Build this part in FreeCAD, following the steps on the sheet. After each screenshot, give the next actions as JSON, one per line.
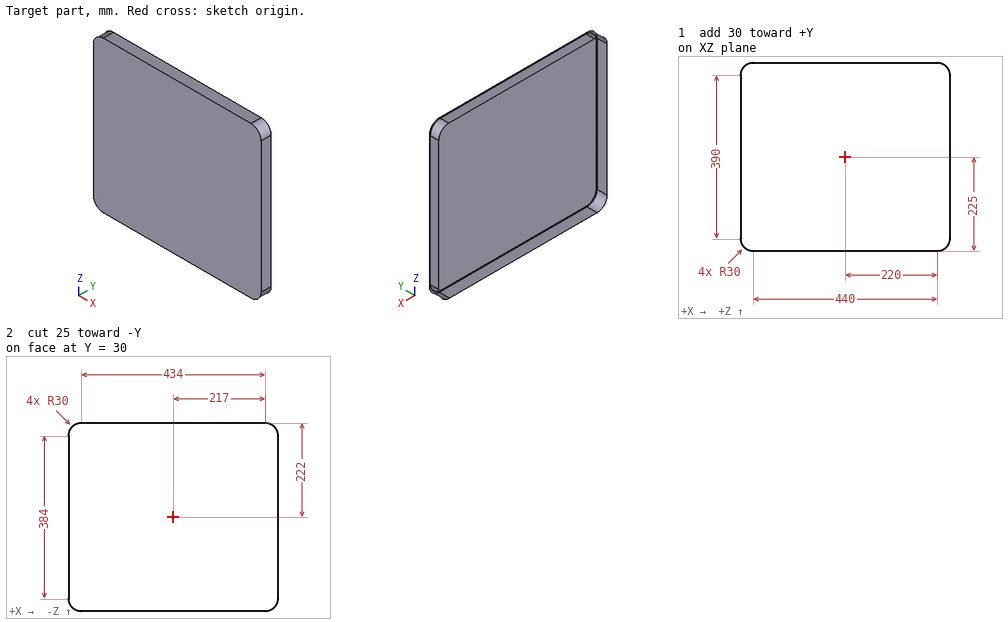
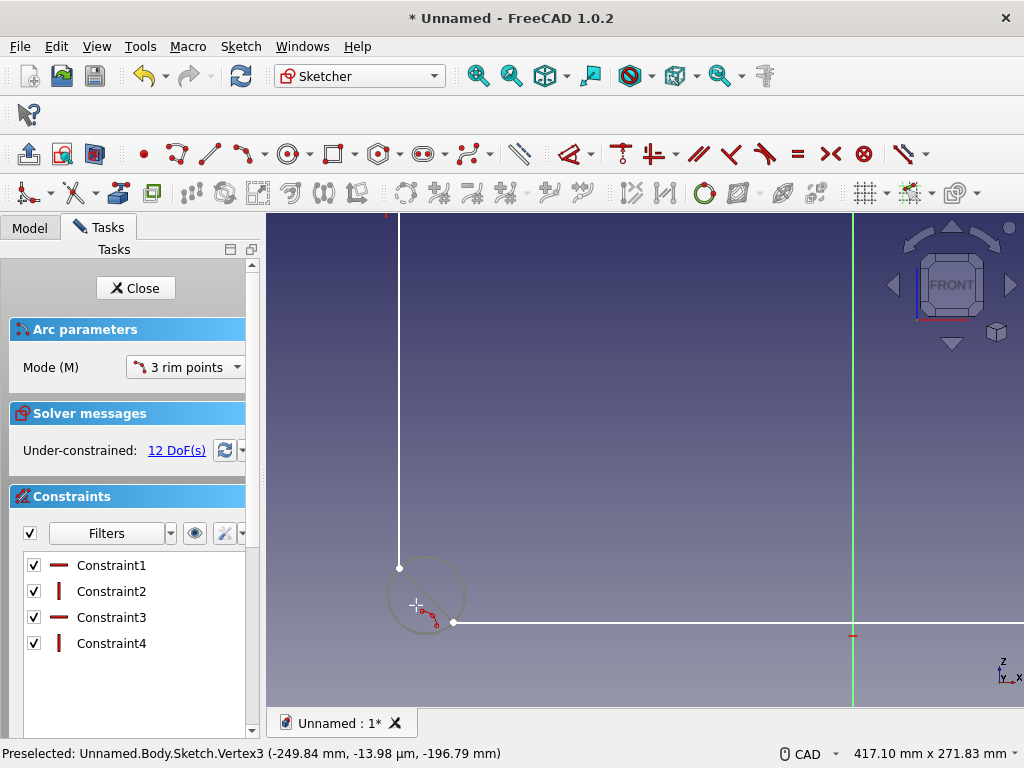
{"action": "left_click", "coordinate": [415, 604]}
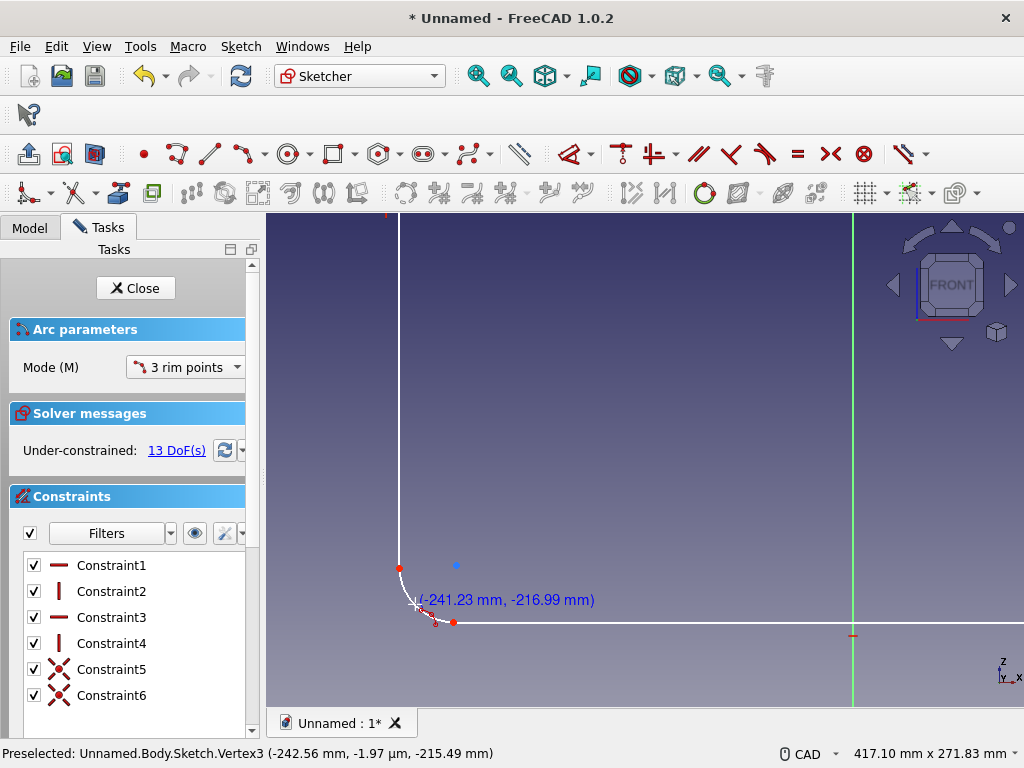
{"action": "scroll", "coordinate": [415, 605], "scroll_direction": "down", "scroll_amount": 5}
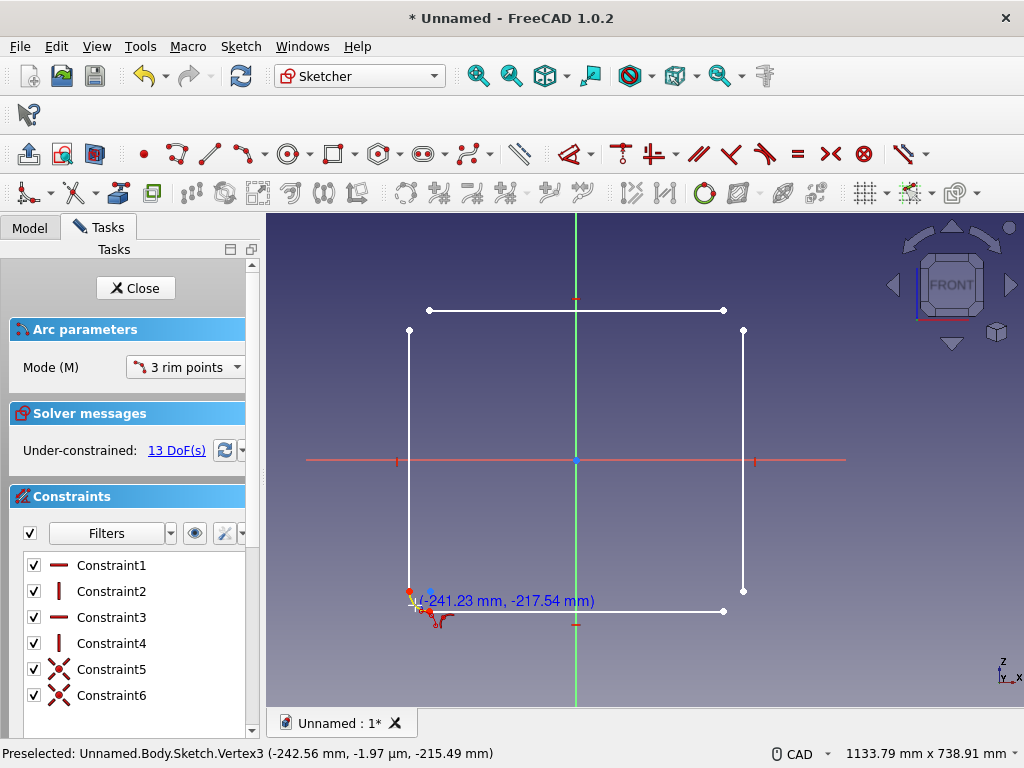
{"action": "left_click", "coordinate": [409, 331]}
{"action": "left_click", "coordinate": [429, 311]}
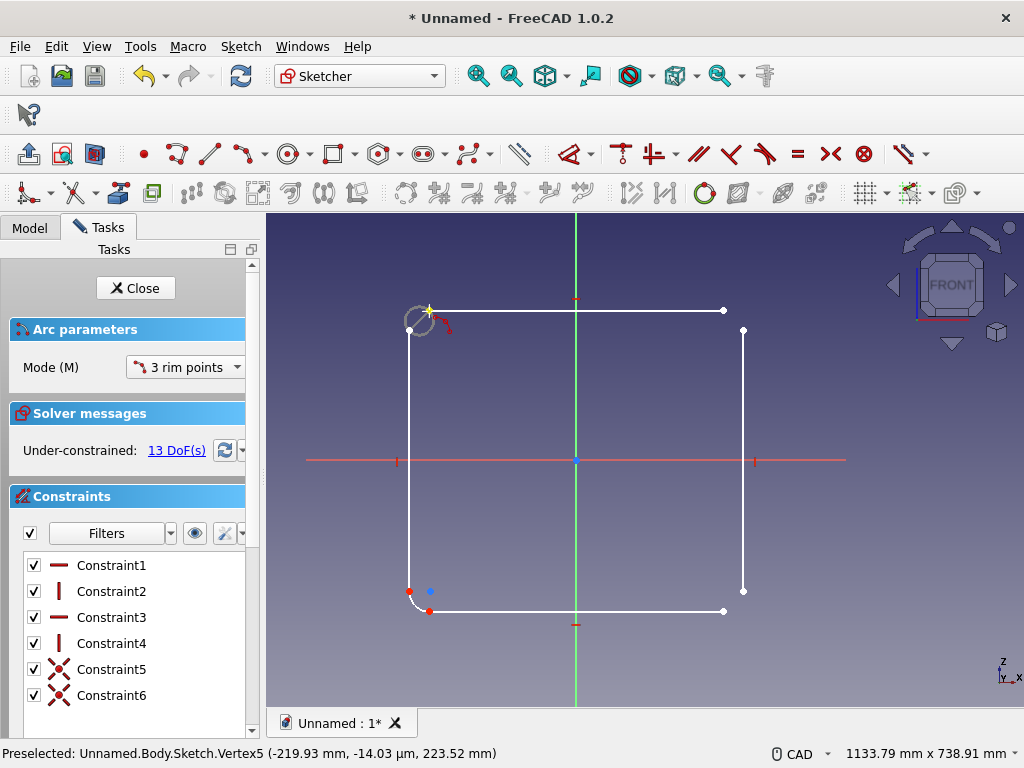
{"action": "scroll", "coordinate": [415, 316], "scroll_direction": "up", "scroll_amount": 5}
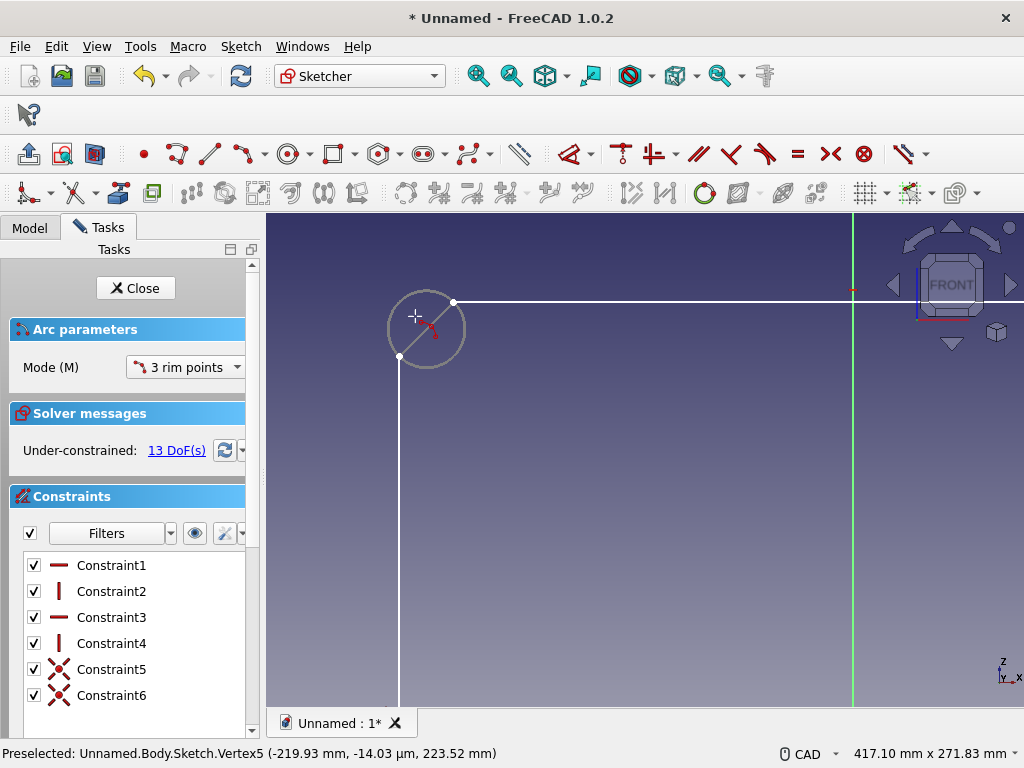
{"action": "left_click", "coordinate": [415, 315]}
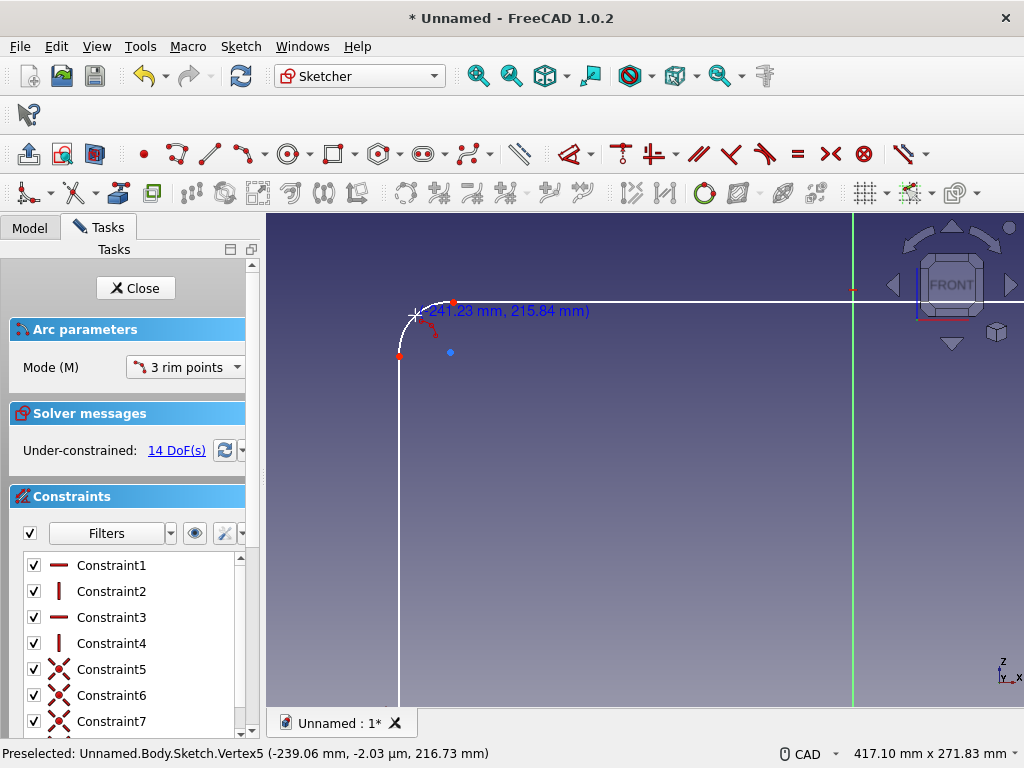
{"action": "scroll", "coordinate": [415, 316], "scroll_direction": "down", "scroll_amount": 5}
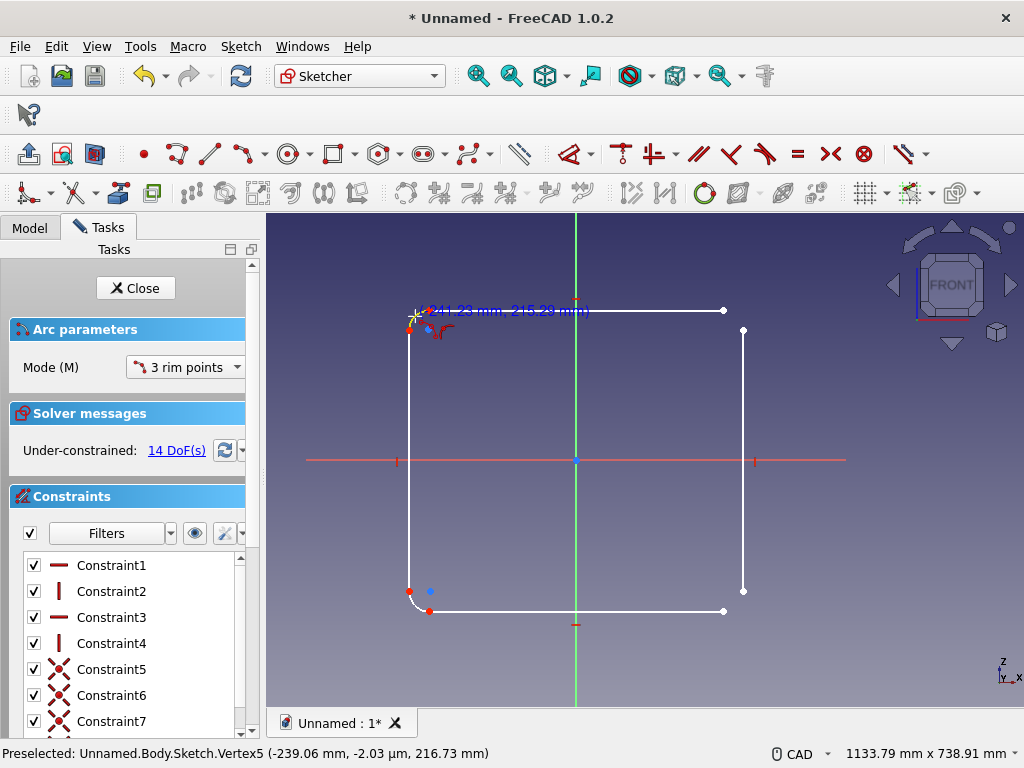
{"action": "left_click", "coordinate": [723, 311]}
{"action": "left_click", "coordinate": [743, 331]}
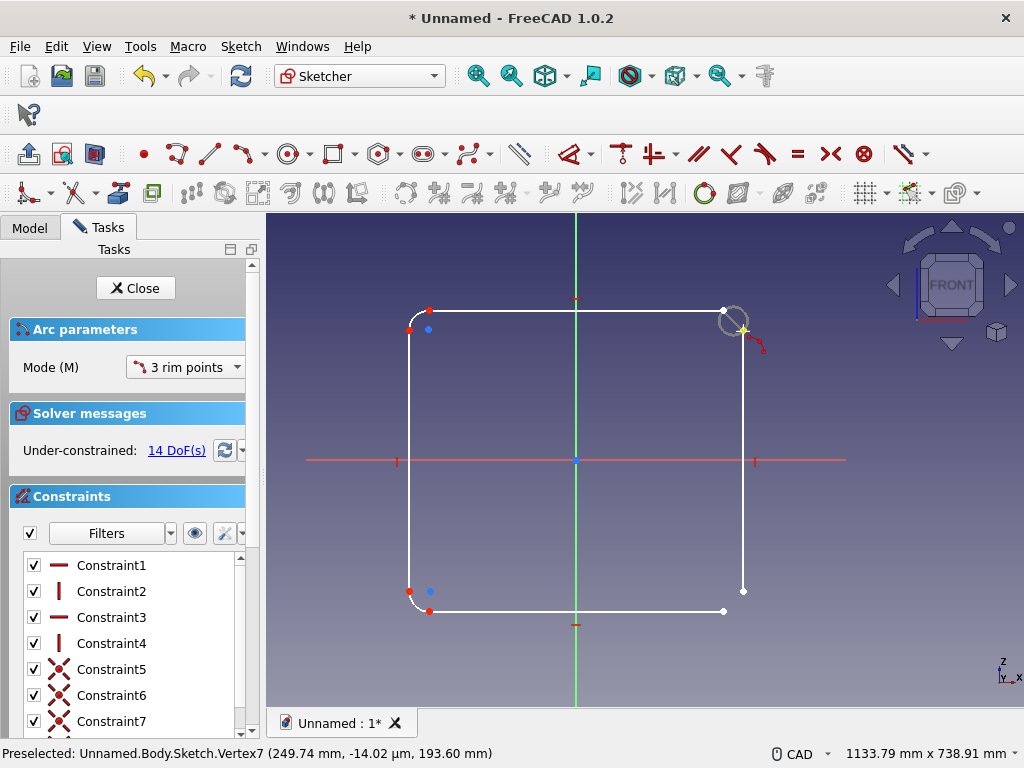
{"action": "scroll", "coordinate": [738, 316], "scroll_direction": "up", "scroll_amount": 5}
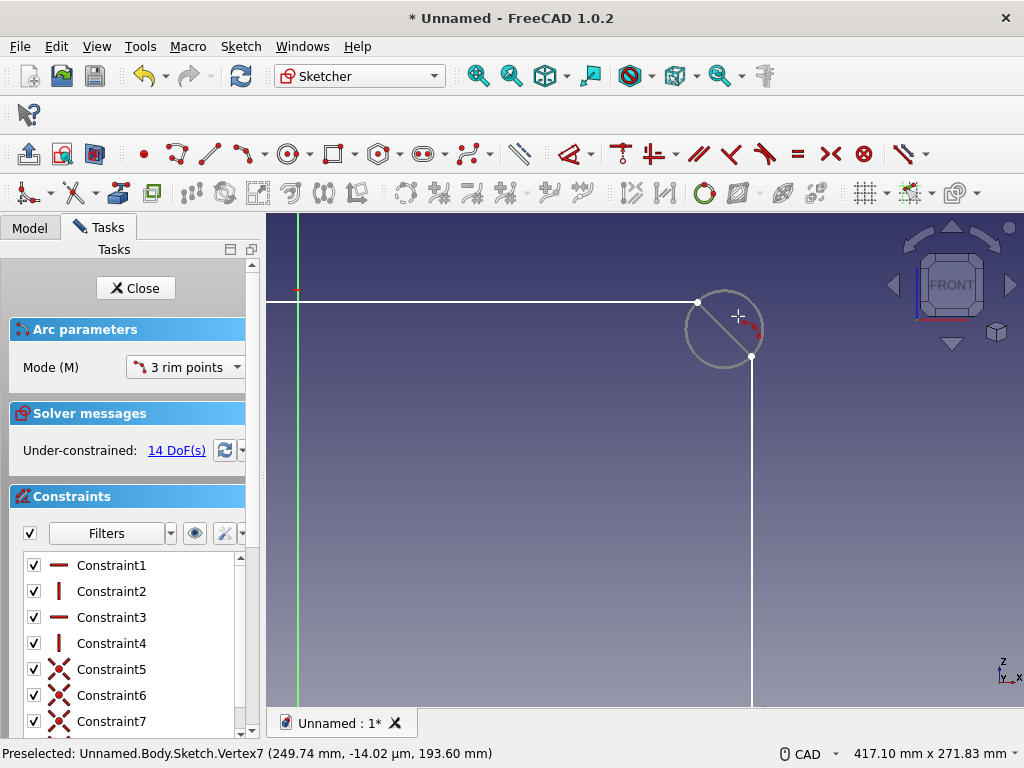
{"action": "left_click", "coordinate": [736, 315]}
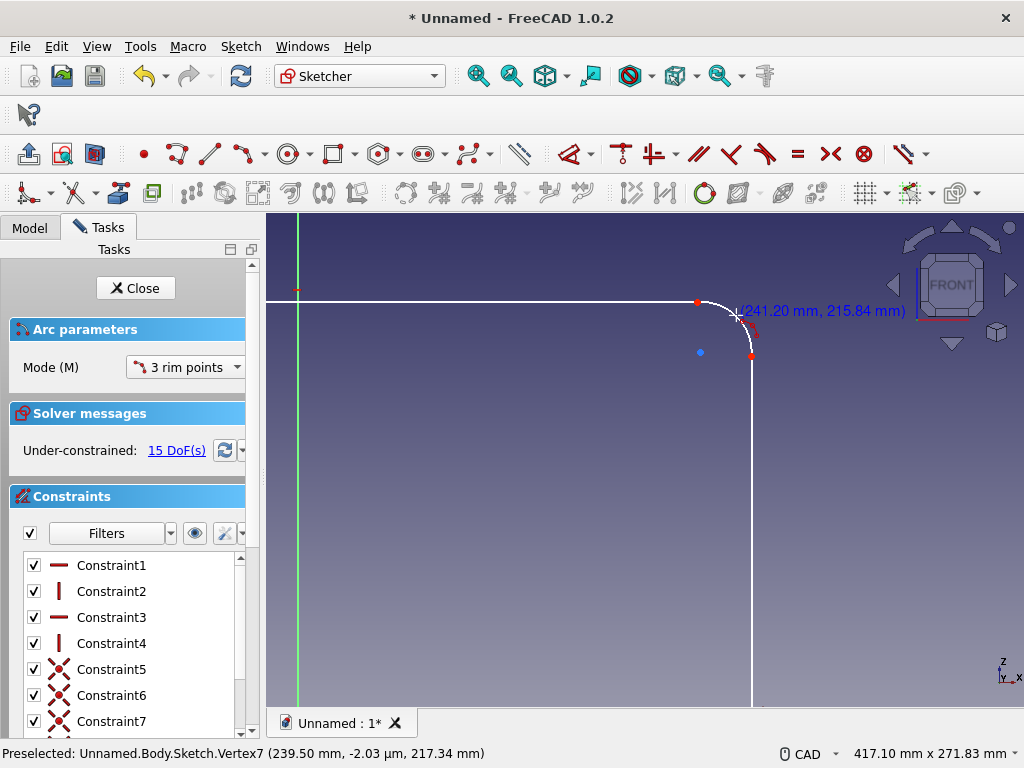
{"action": "scroll", "coordinate": [739, 316], "scroll_direction": "down", "scroll_amount": 5}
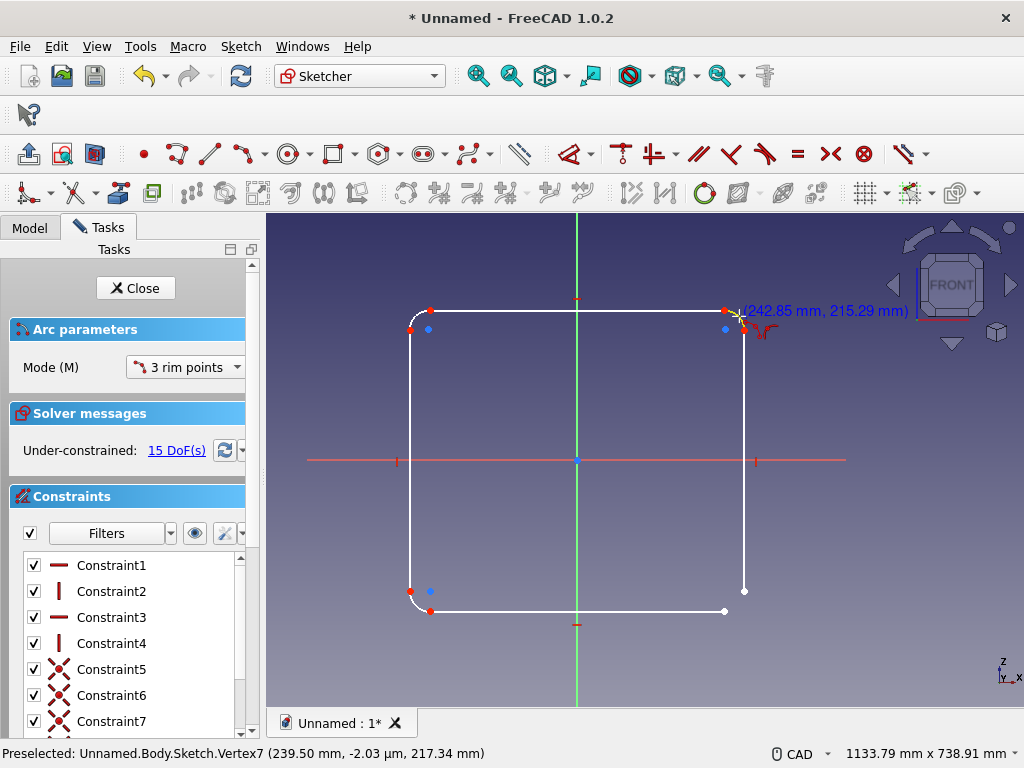
{"action": "left_click", "coordinate": [744, 592]}
{"action": "left_click", "coordinate": [724, 612]}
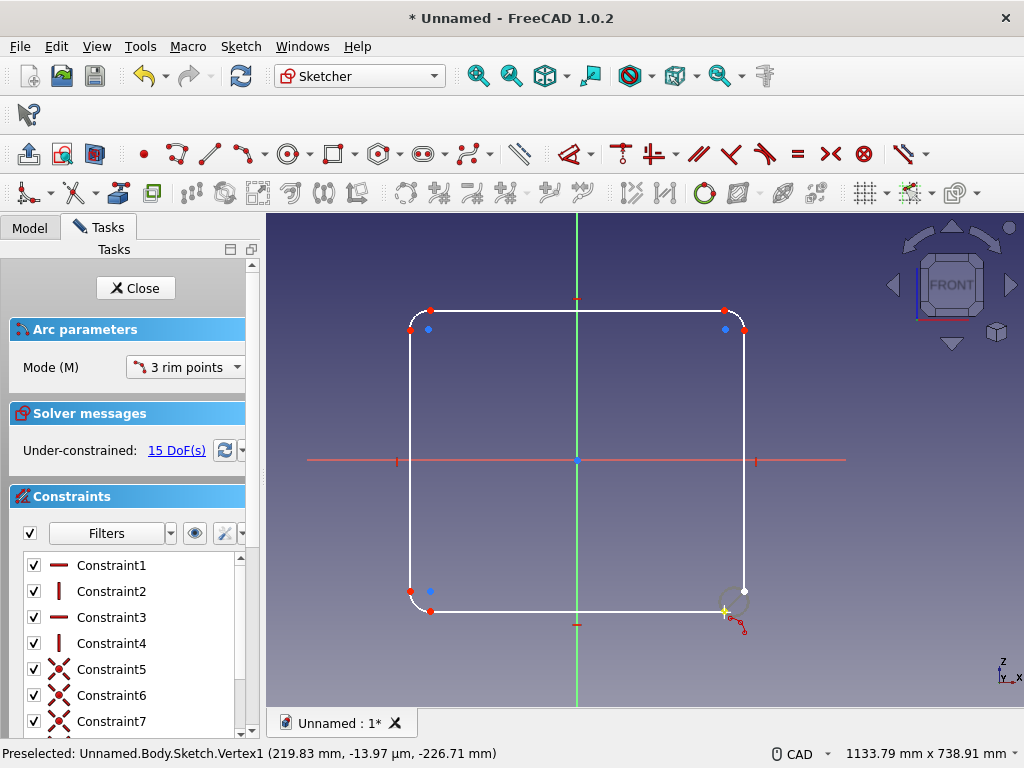
{"action": "scroll", "coordinate": [738, 605], "scroll_direction": "up", "scroll_amount": 5}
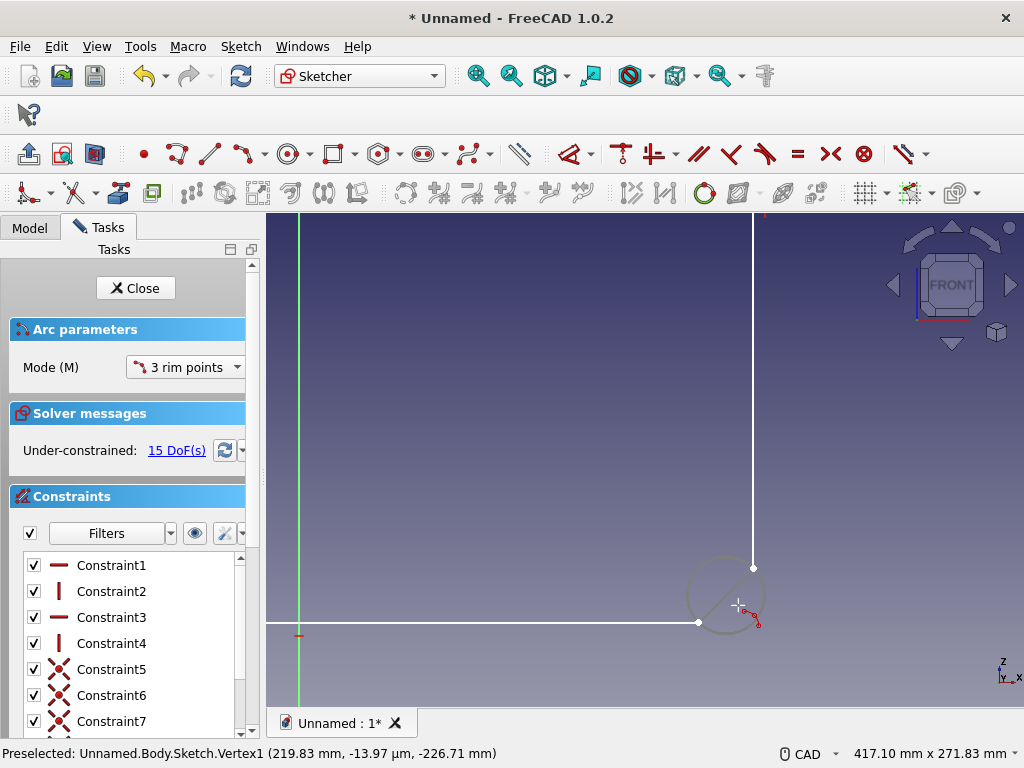
{"action": "left_click", "coordinate": [738, 604]}
{"action": "key", "text": "Escape"}